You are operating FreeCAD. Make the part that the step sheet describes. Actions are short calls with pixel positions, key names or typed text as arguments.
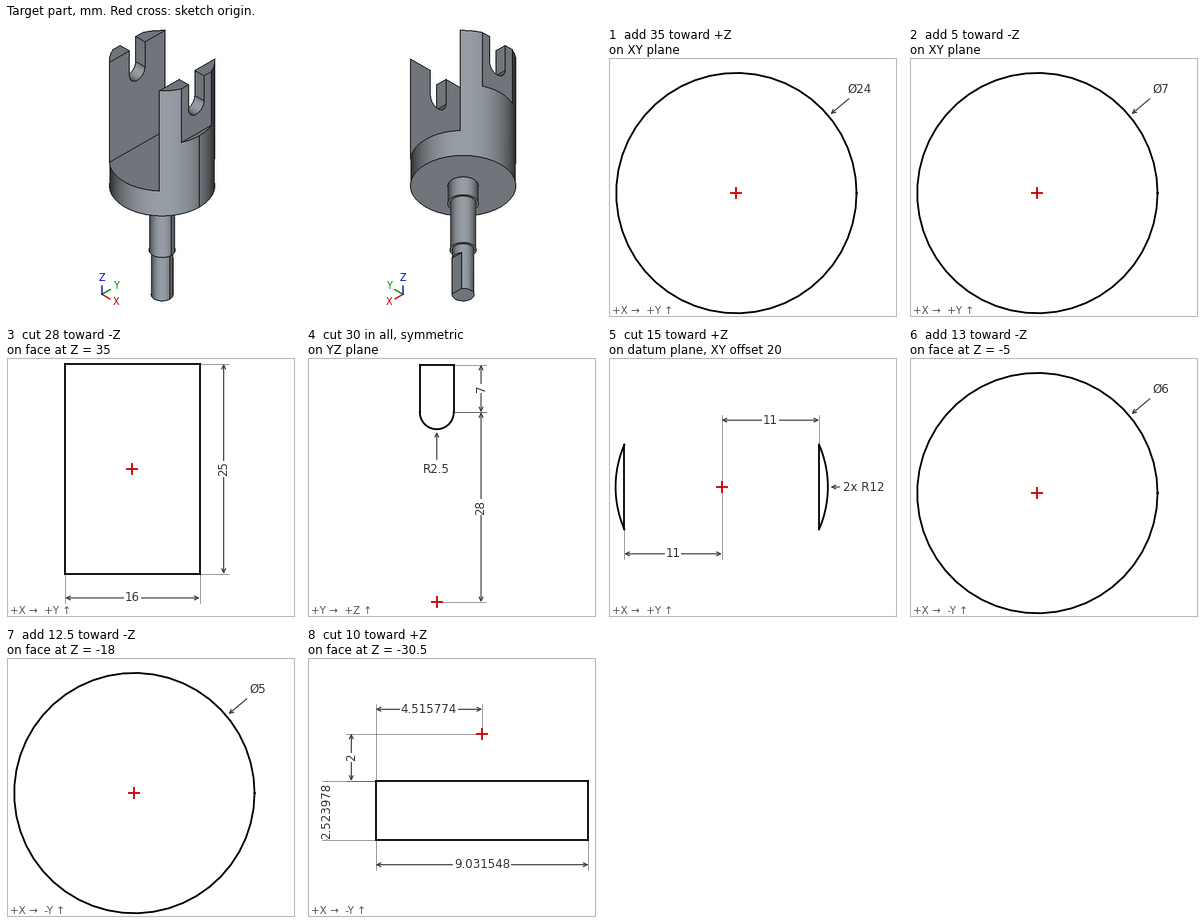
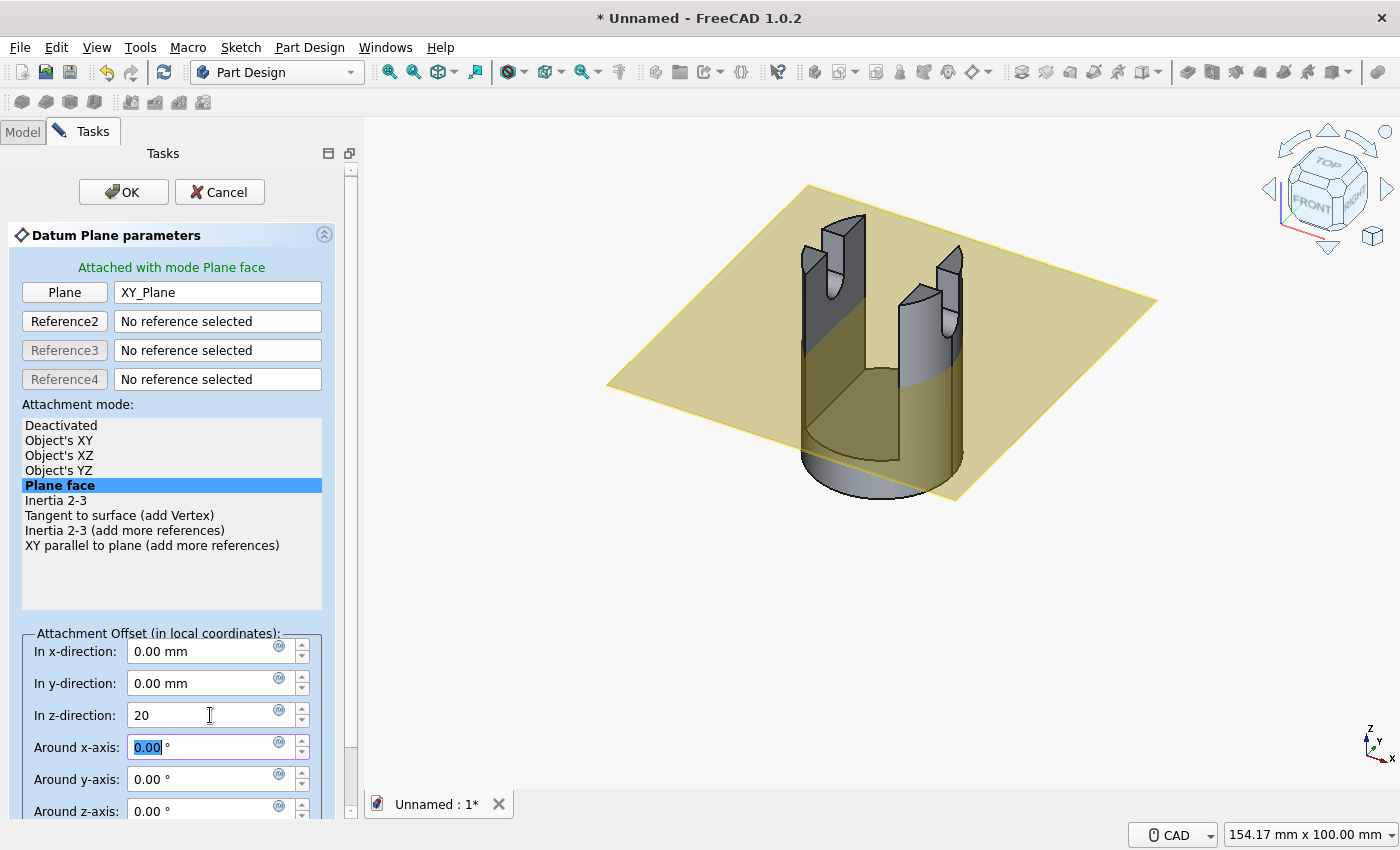
click(124, 192)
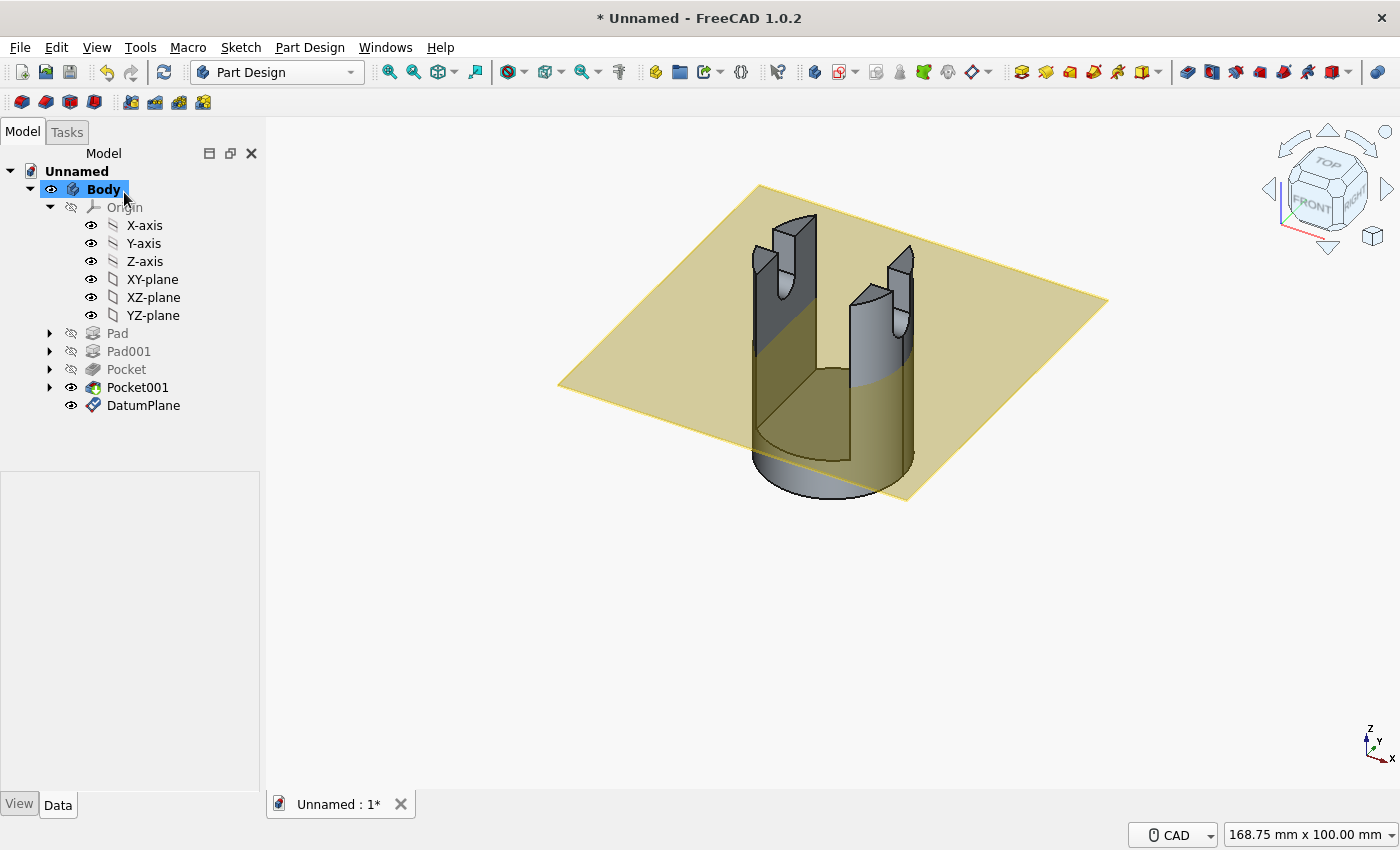
click(116, 405)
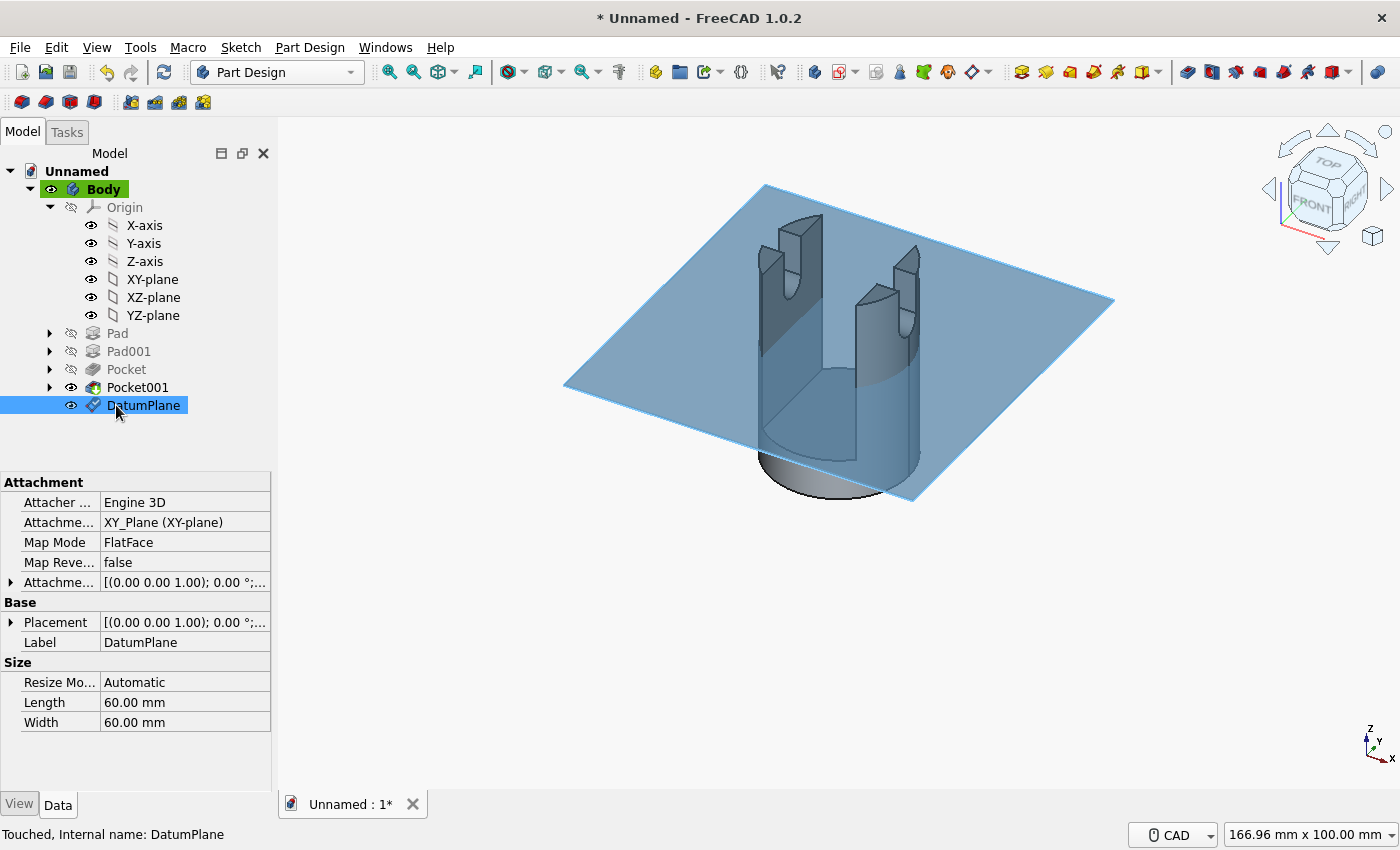
click(840, 72)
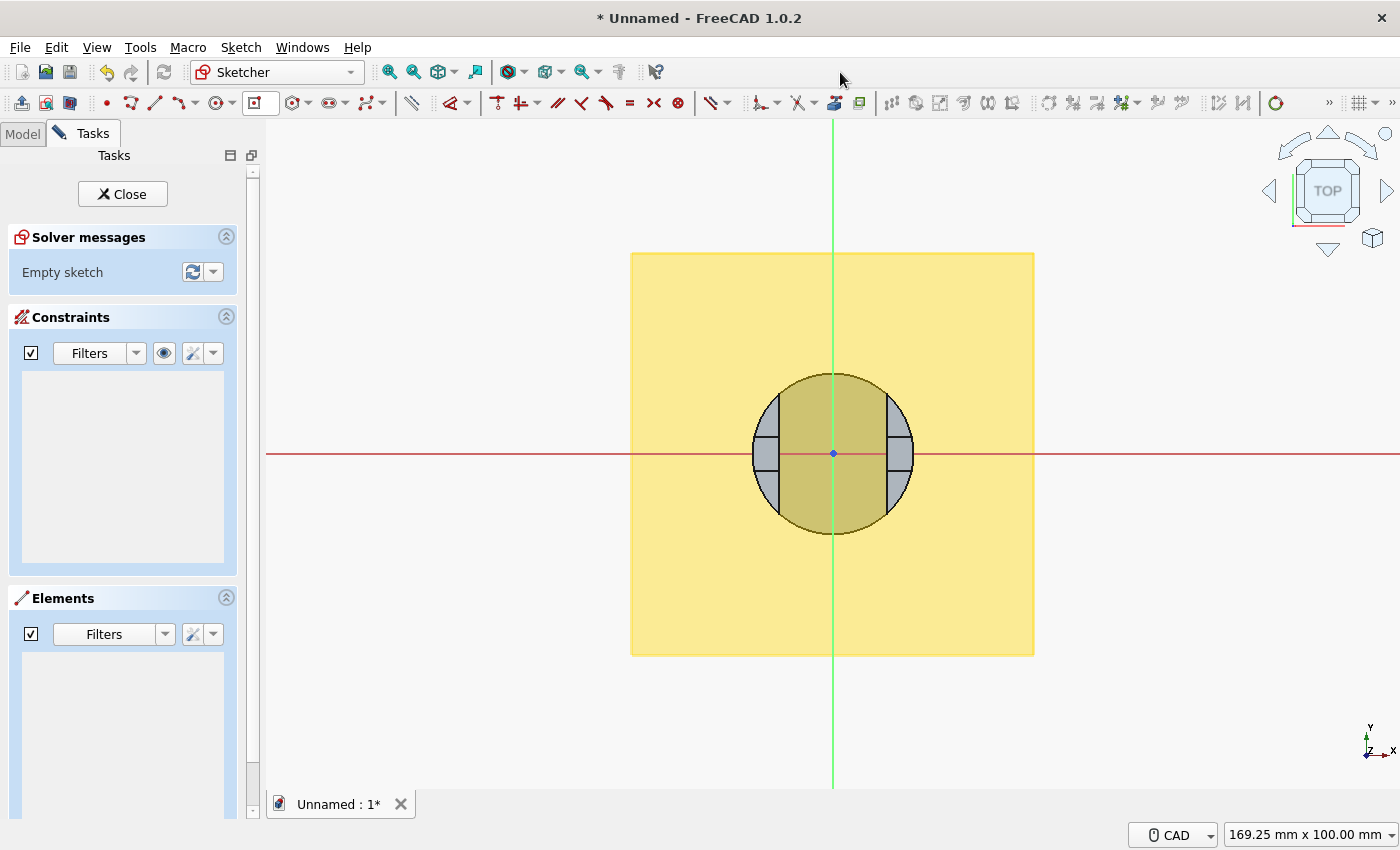
click(70, 104)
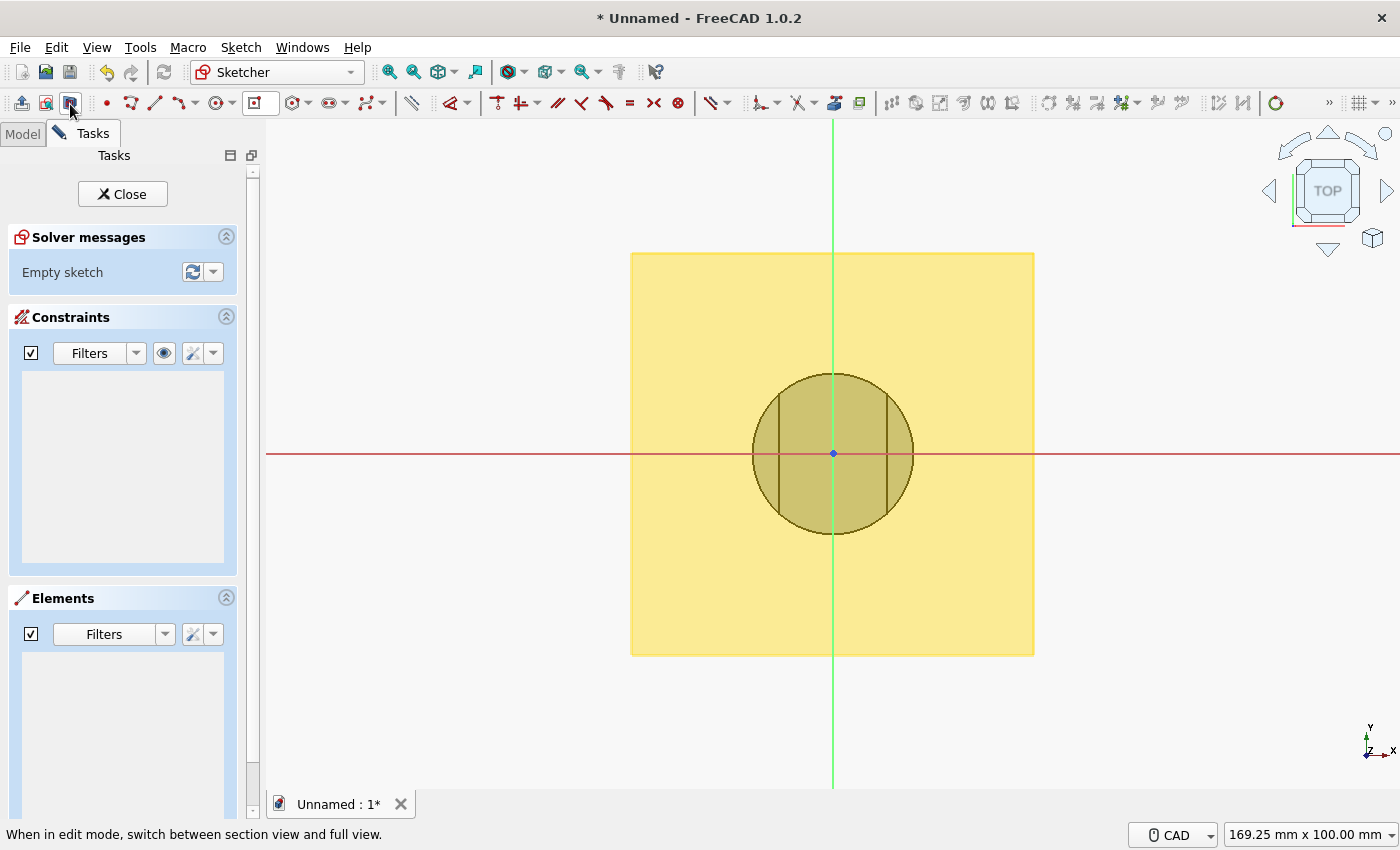
scroll(855, 454, up, 7)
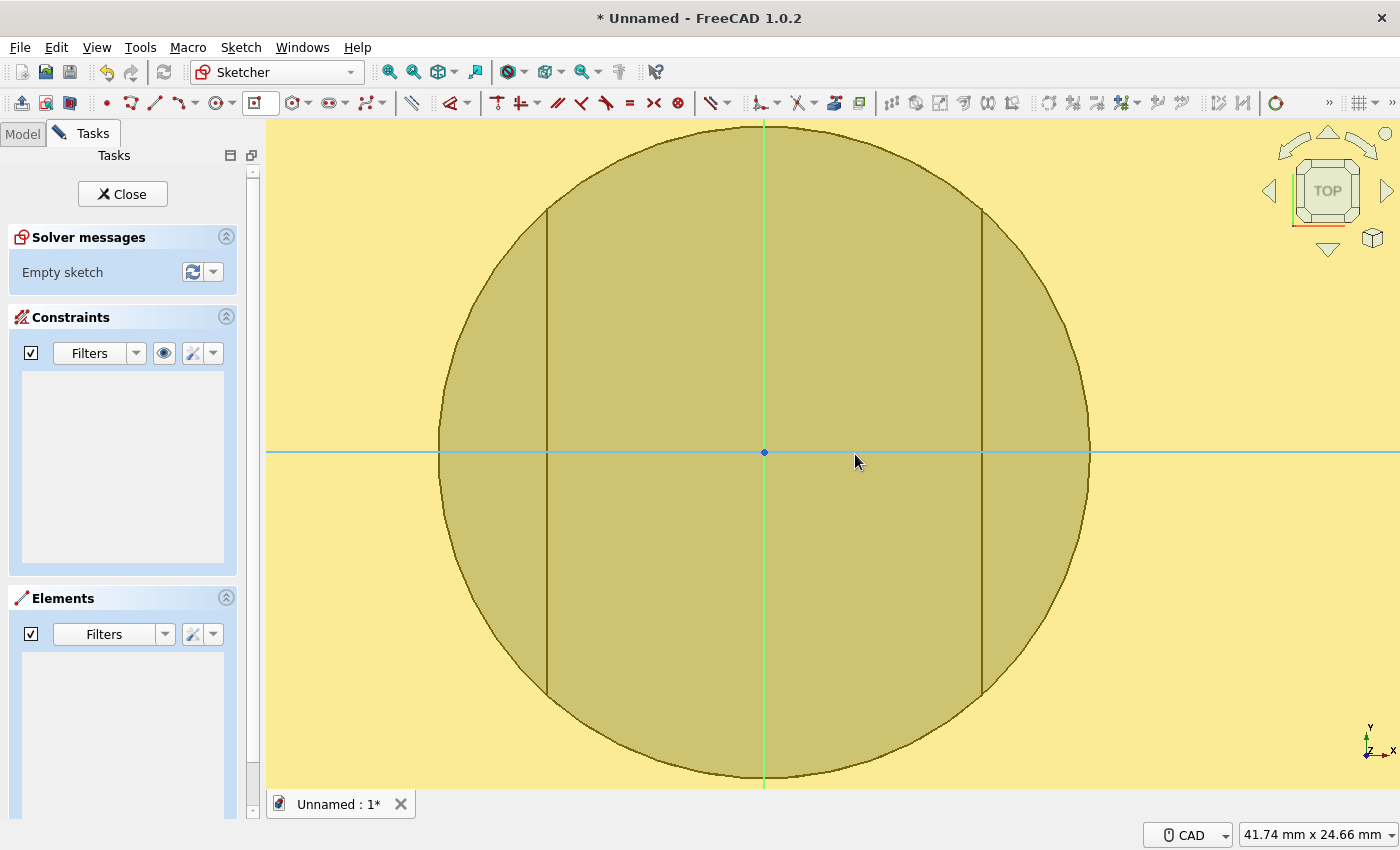
click(156, 104)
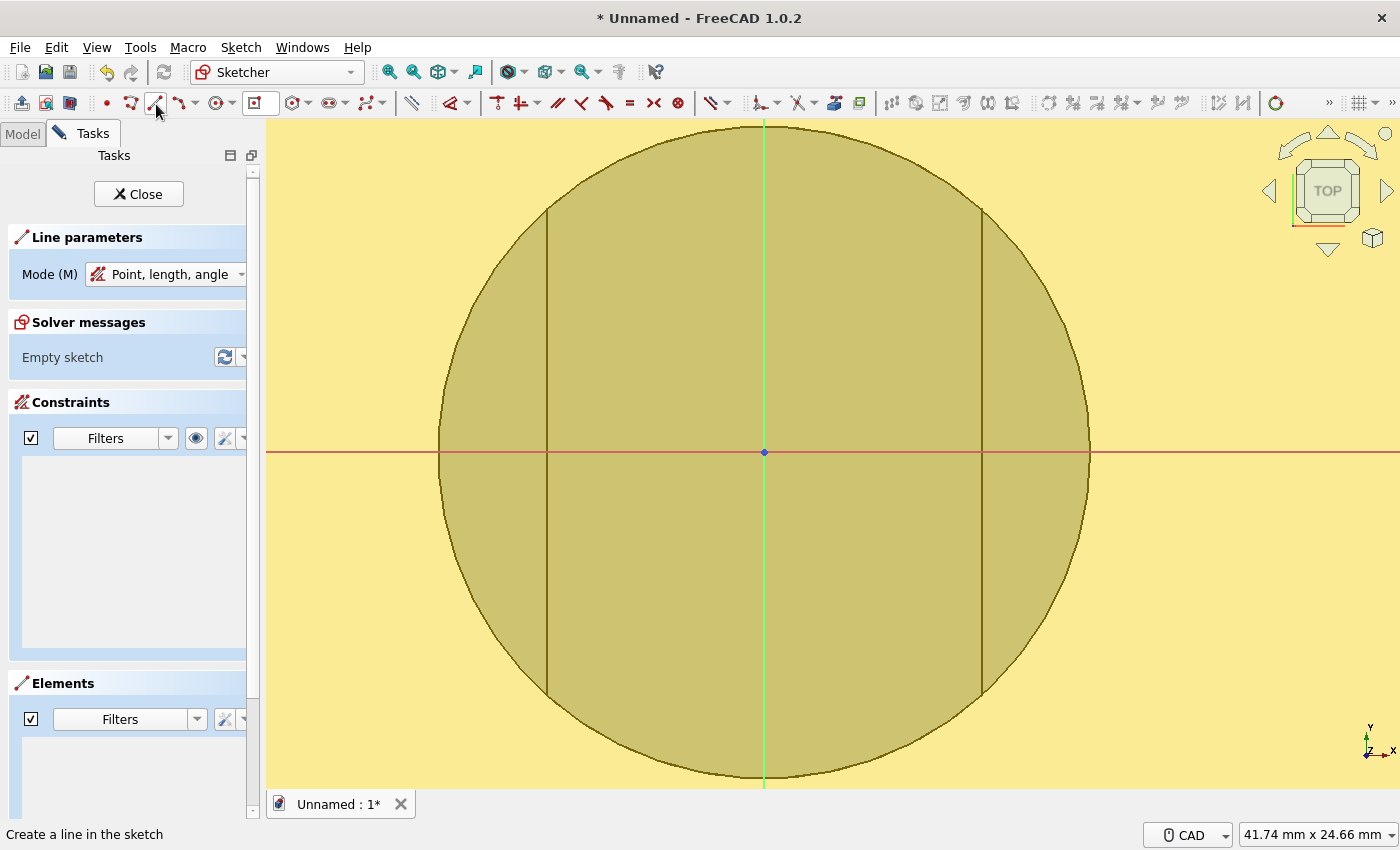
click(1063, 322)
click(1063, 583)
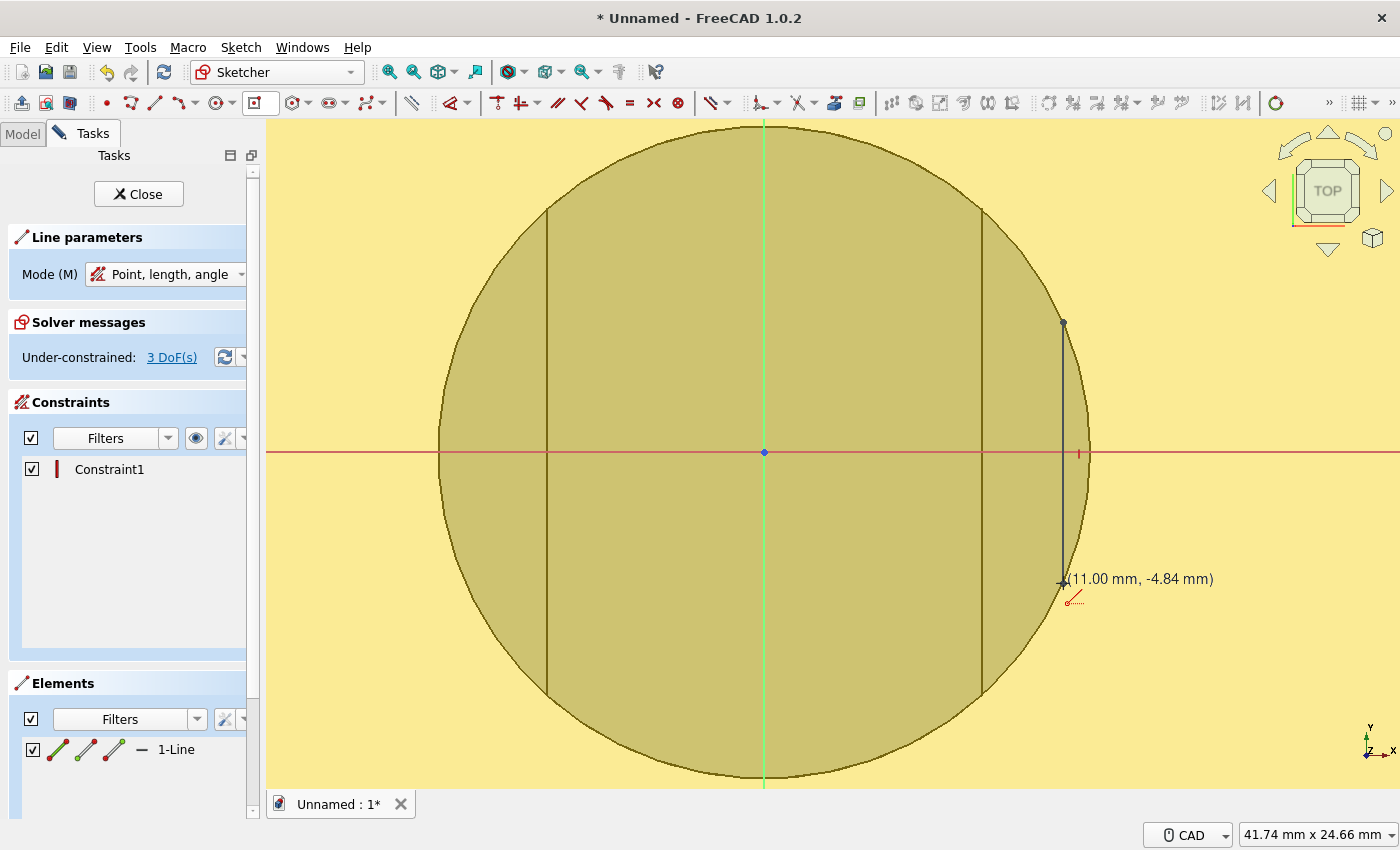
click(180, 104)